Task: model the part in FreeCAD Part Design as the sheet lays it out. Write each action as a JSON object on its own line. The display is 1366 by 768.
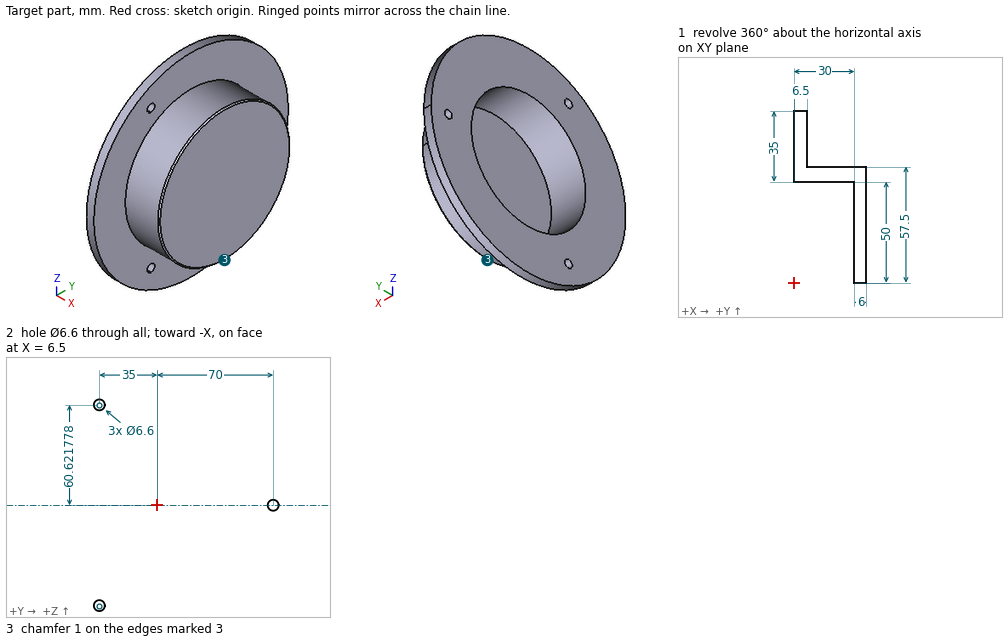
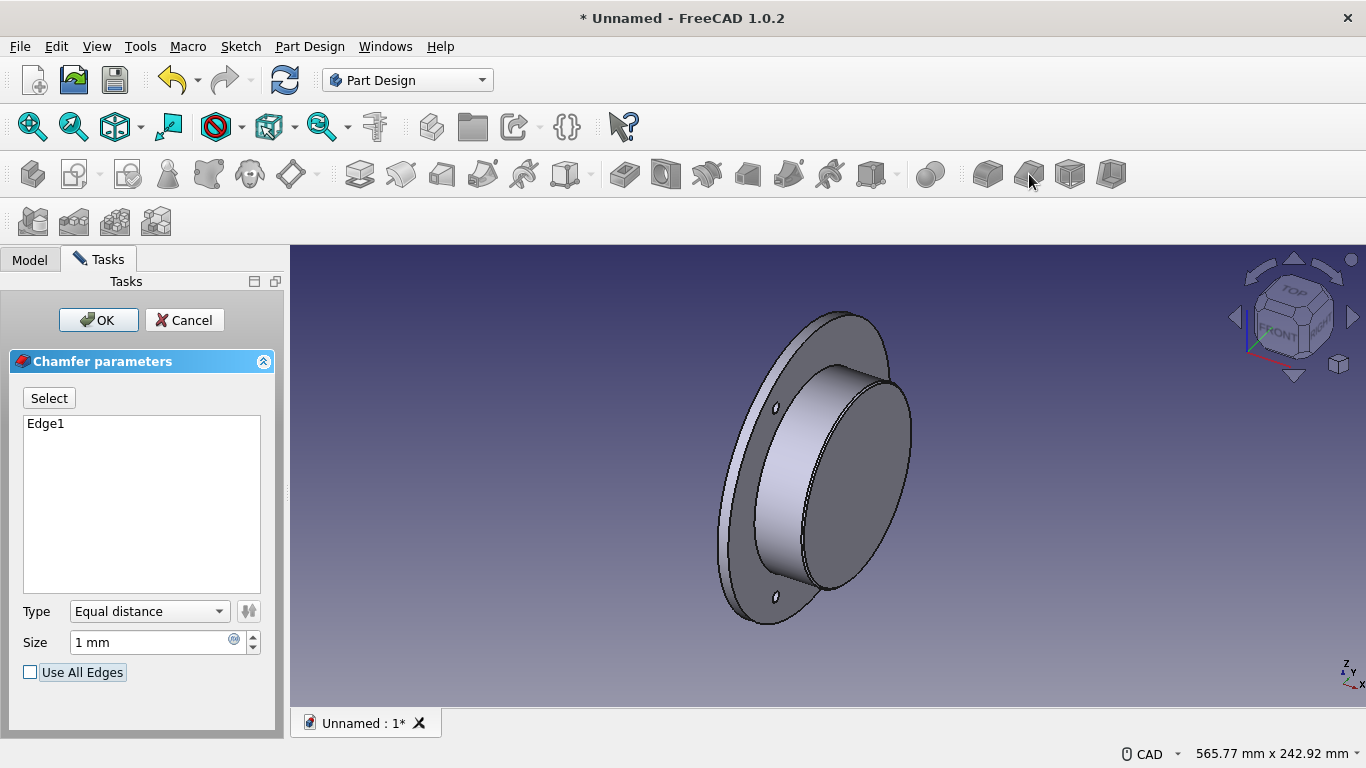
{"action": "left_click", "coordinate": [99, 320]}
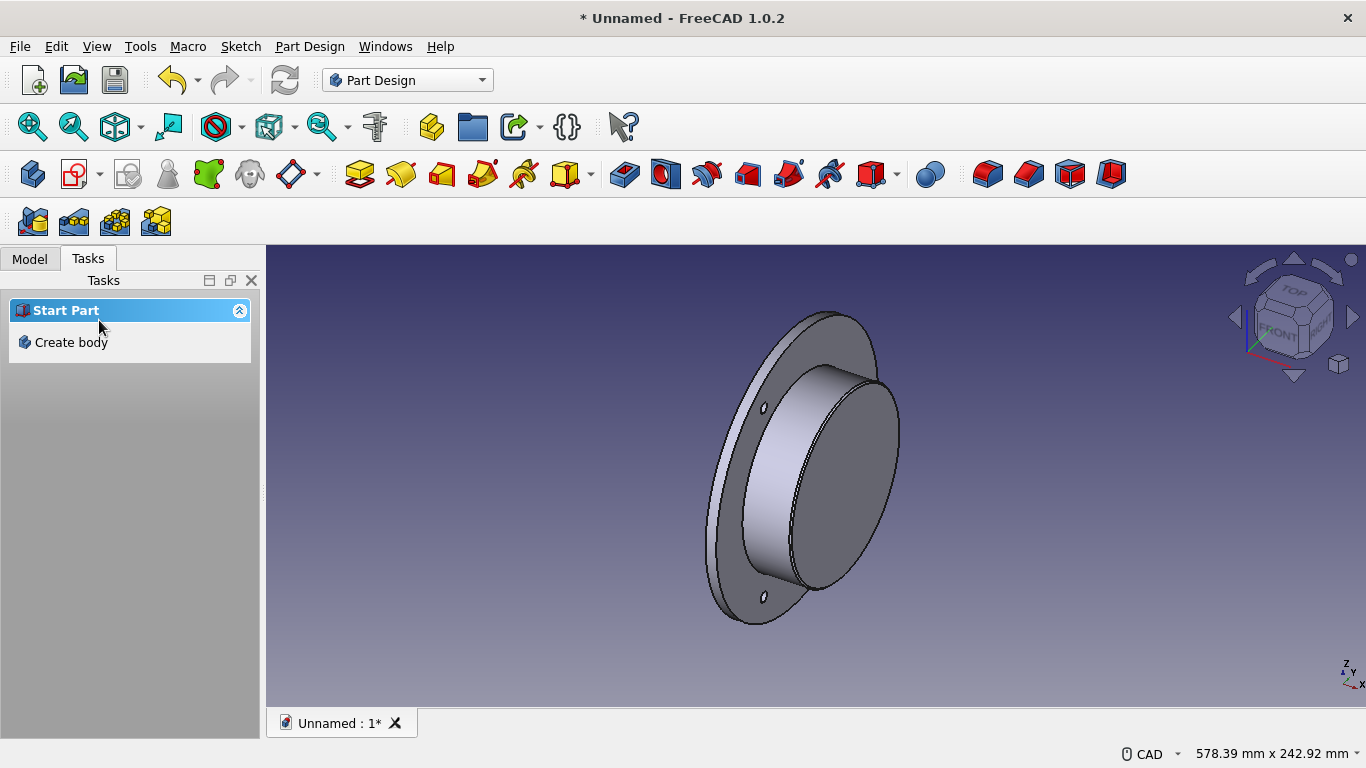
{"action": "key", "text": "0"}